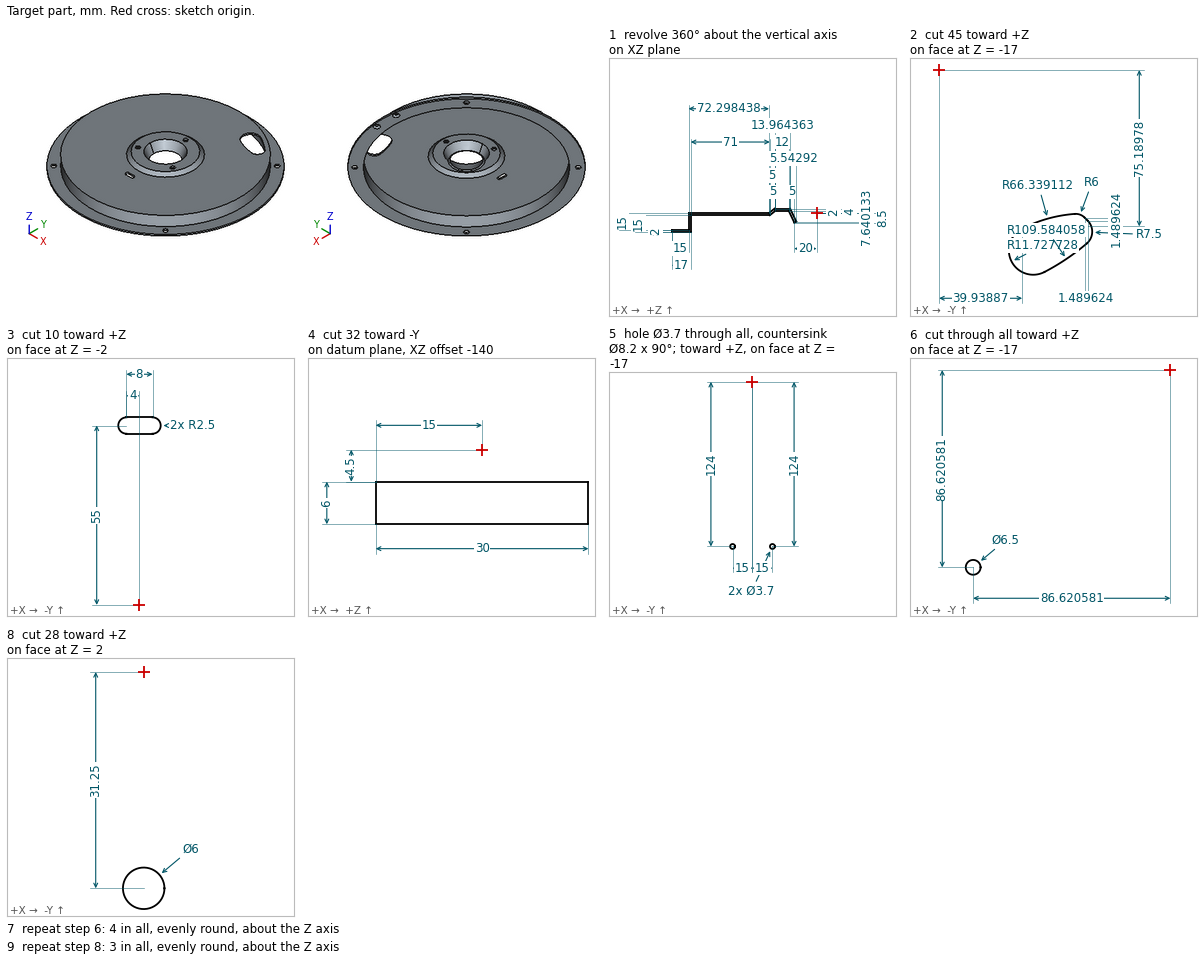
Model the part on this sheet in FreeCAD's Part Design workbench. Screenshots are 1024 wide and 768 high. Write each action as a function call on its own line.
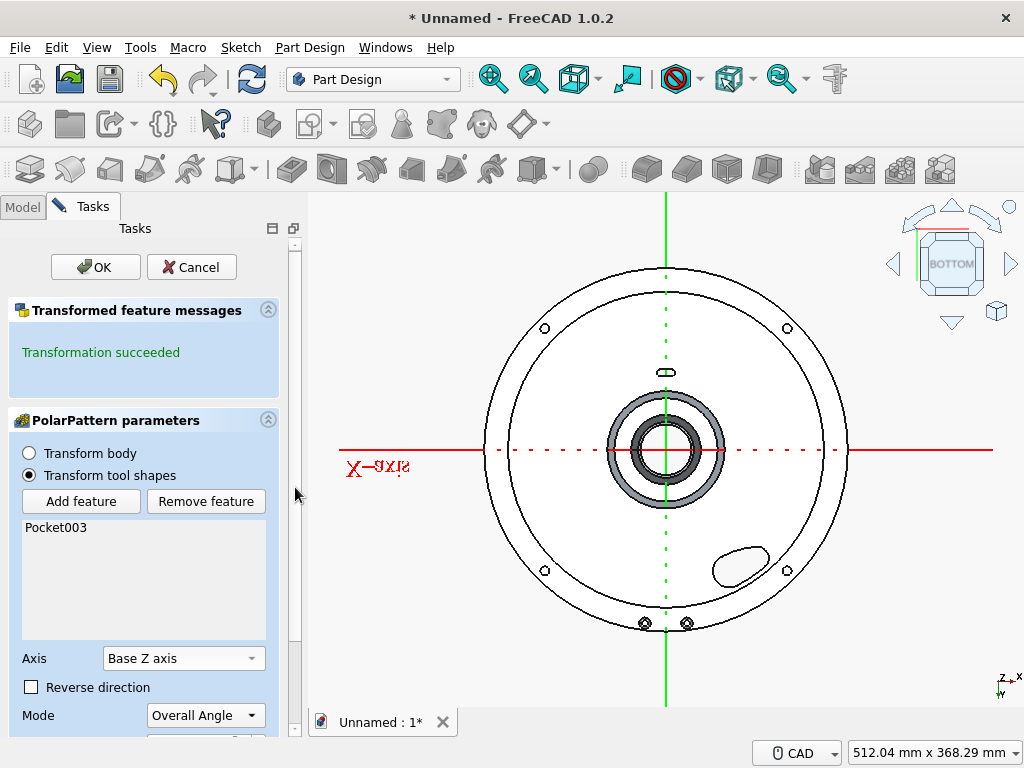
click(96, 267)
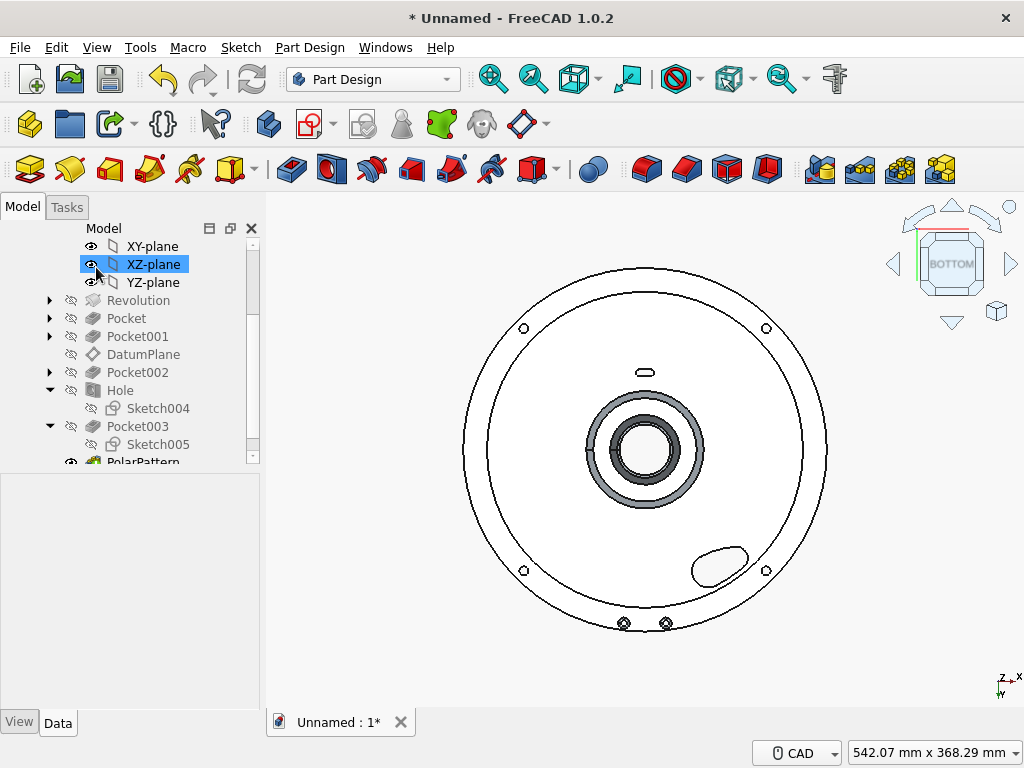
click(645, 493)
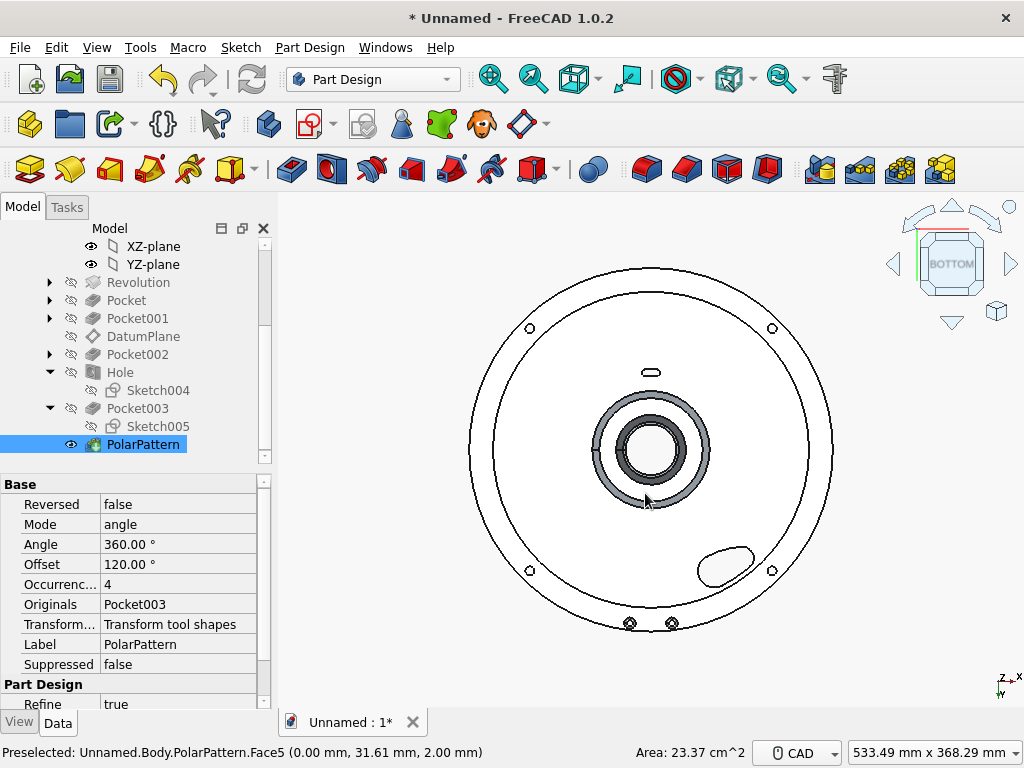
click(310, 124)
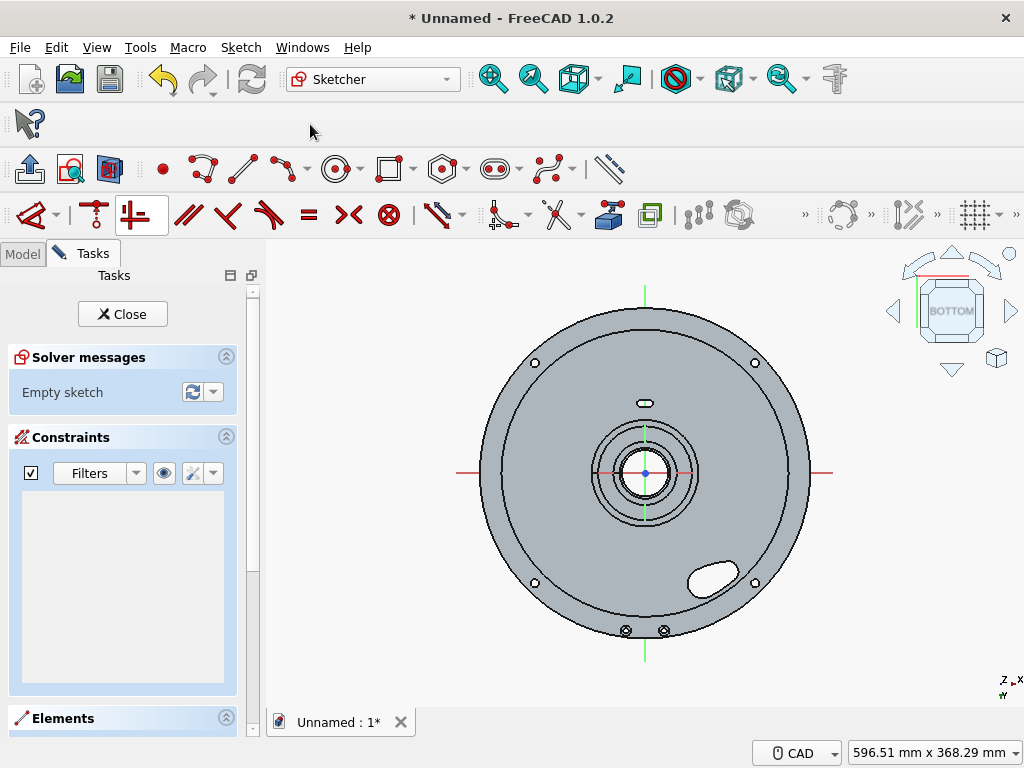
scroll(649, 515, up, 15)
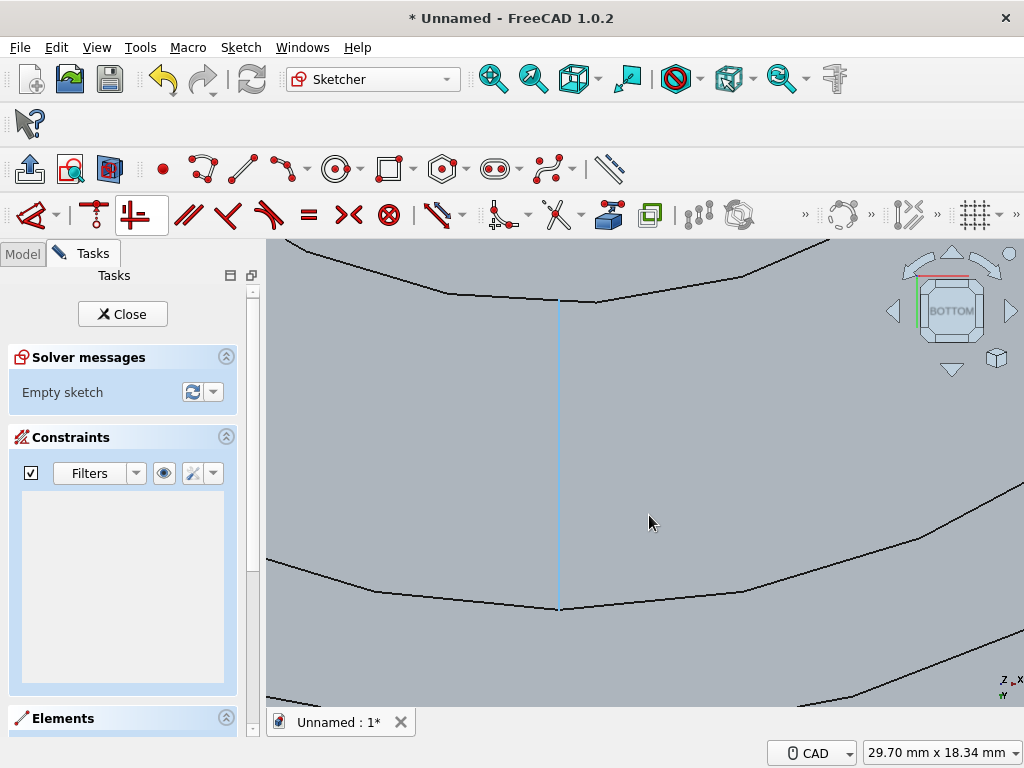
scroll(538, 451, up, 3)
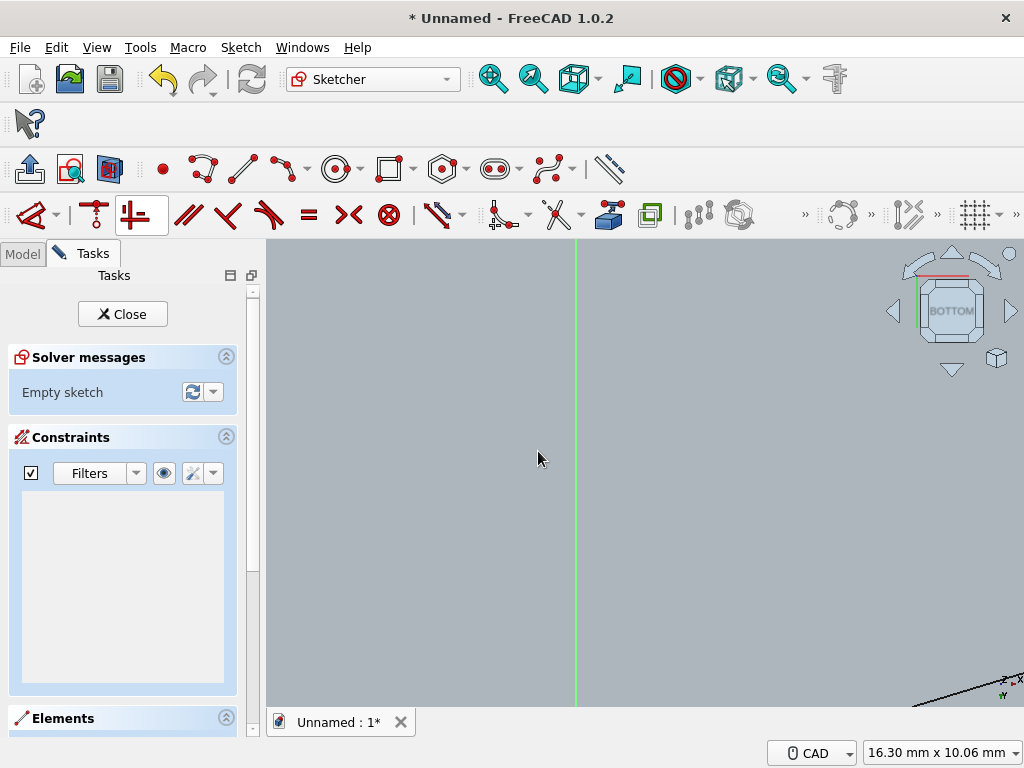
click(336, 170)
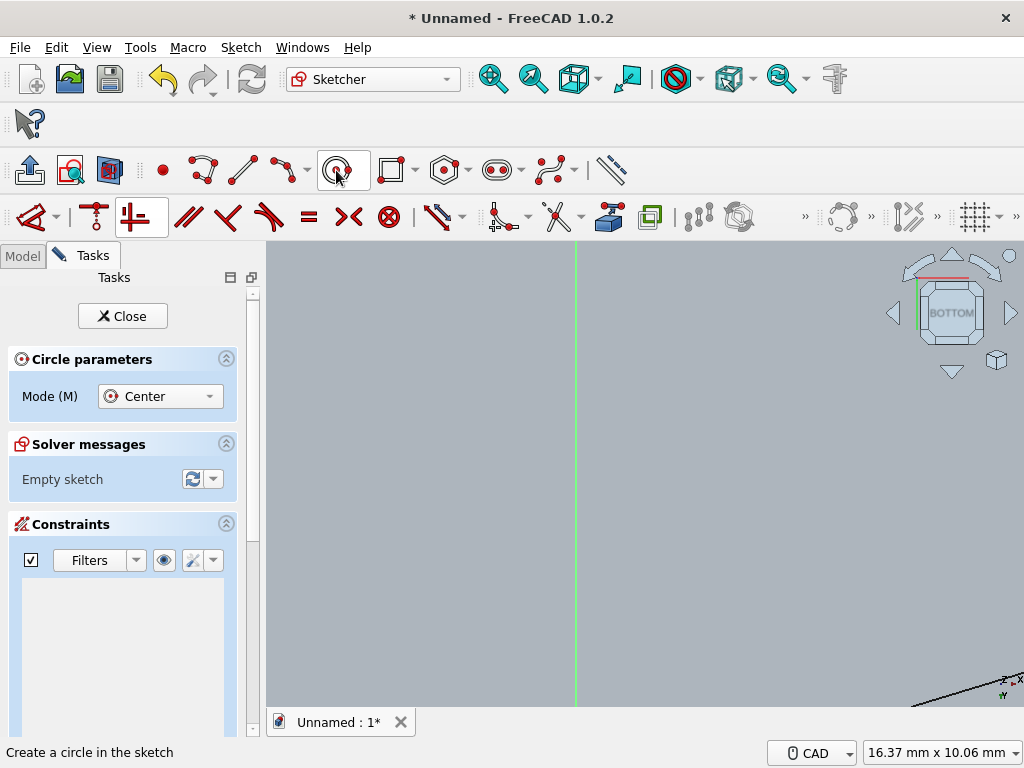
click(576, 474)
click(675, 376)
key(Escape)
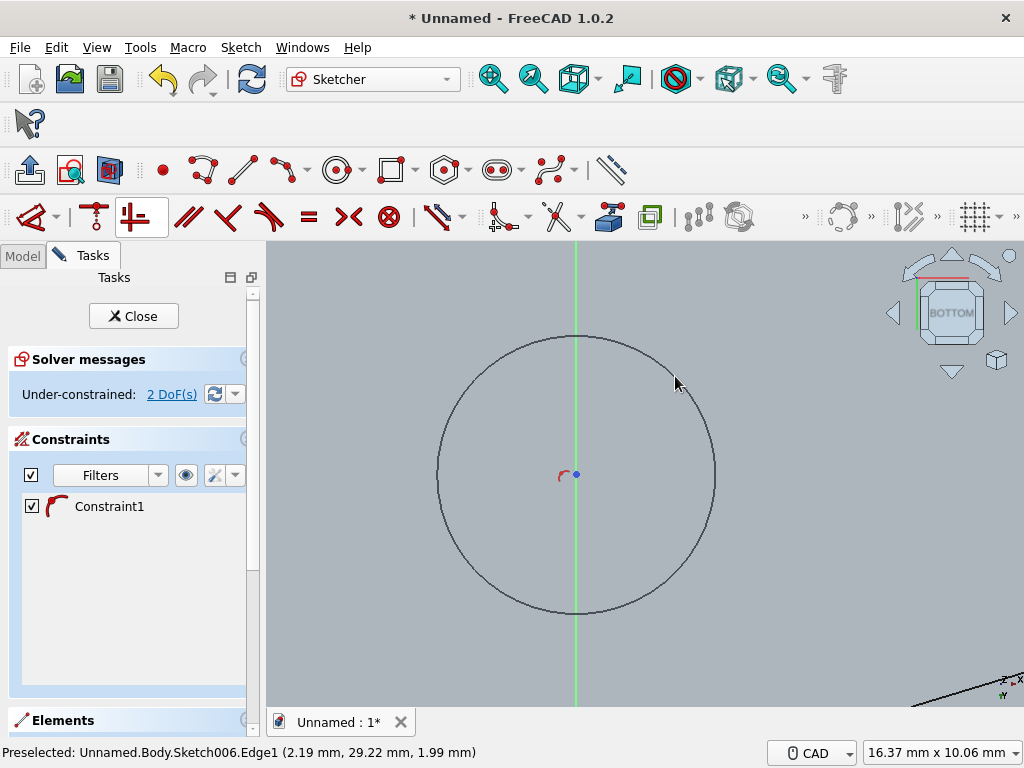
click(32, 218)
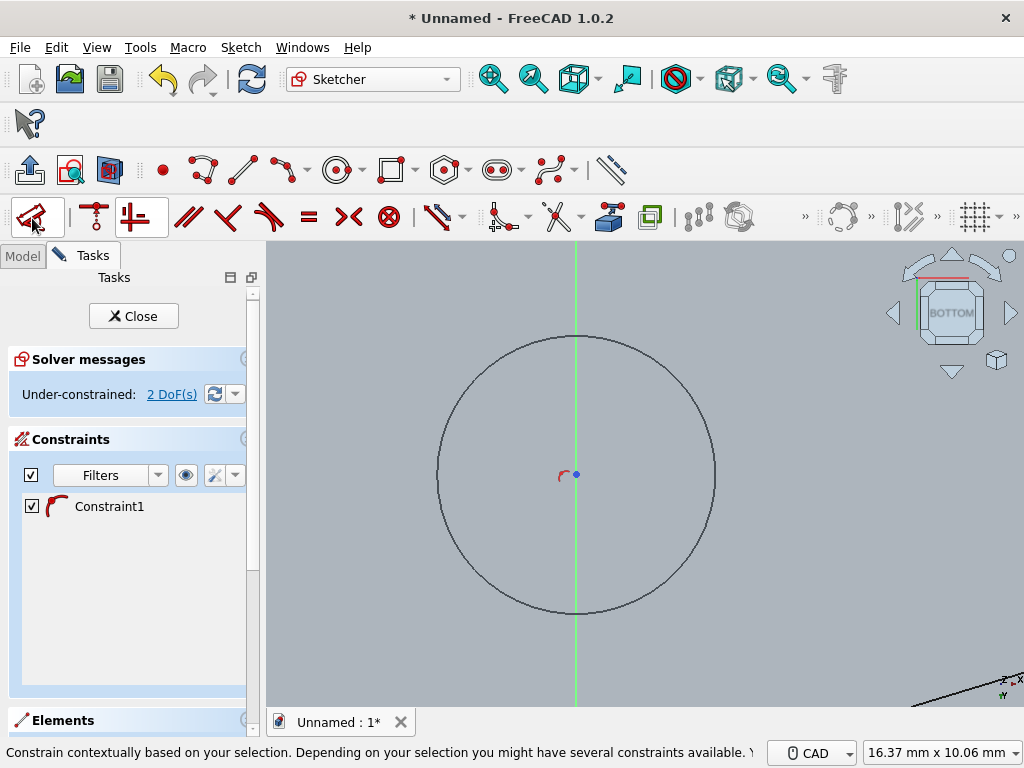
click(674, 376)
click(696, 353)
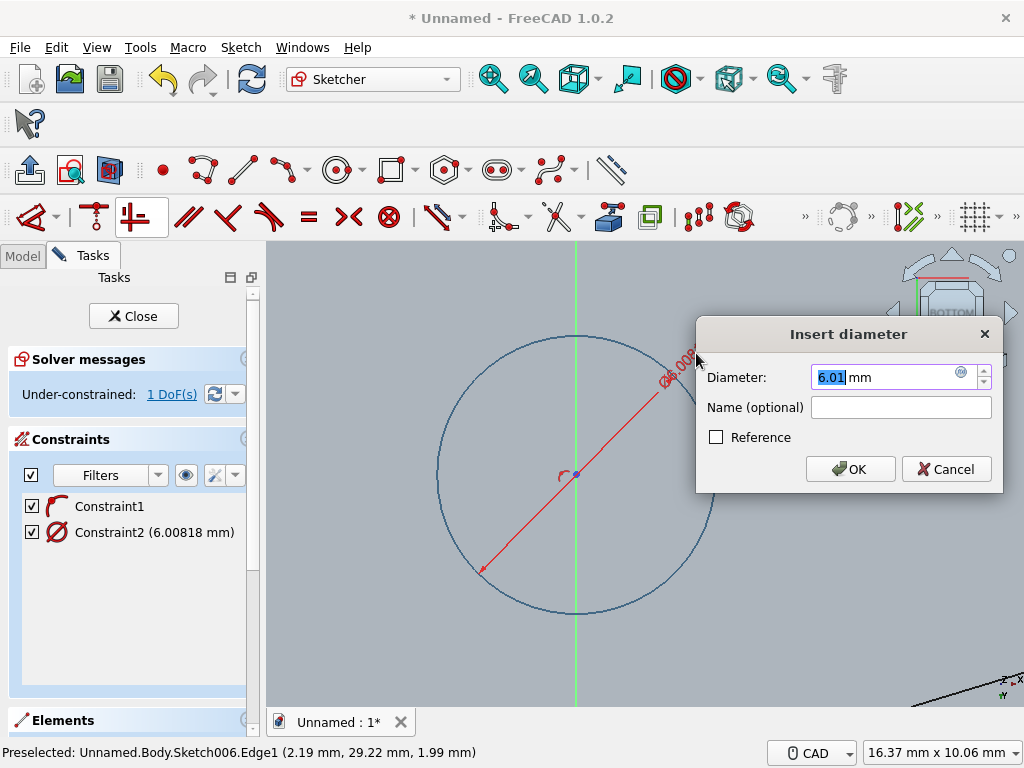
text(6)
key(Return)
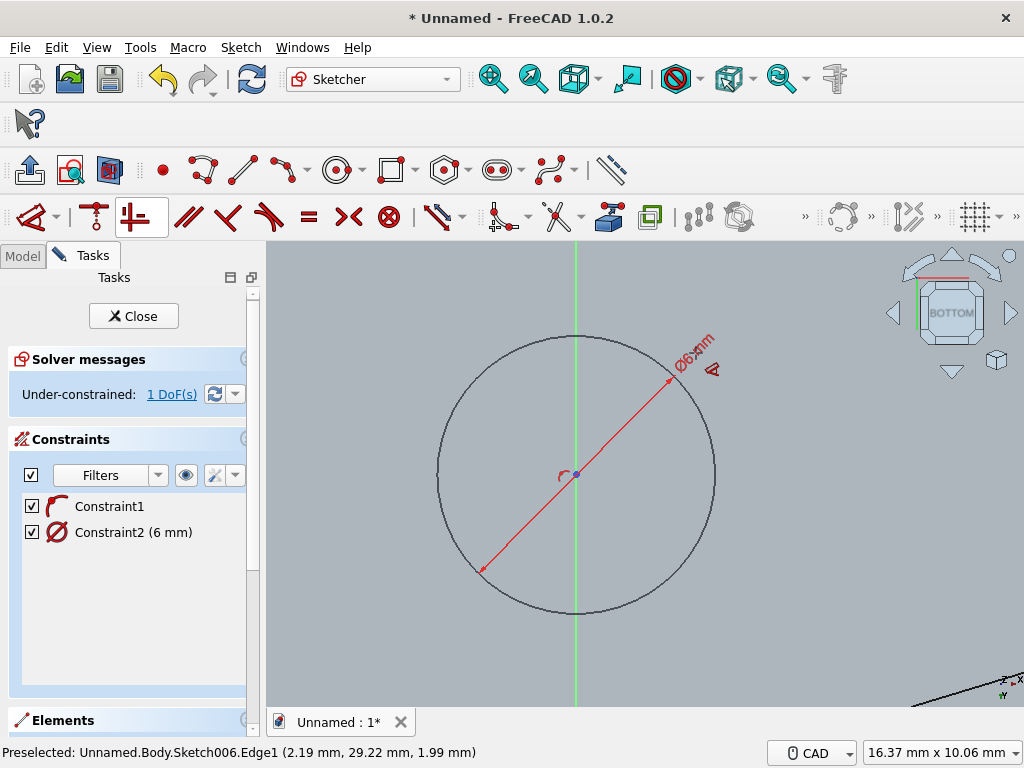
click(576, 475)
click(610, 372)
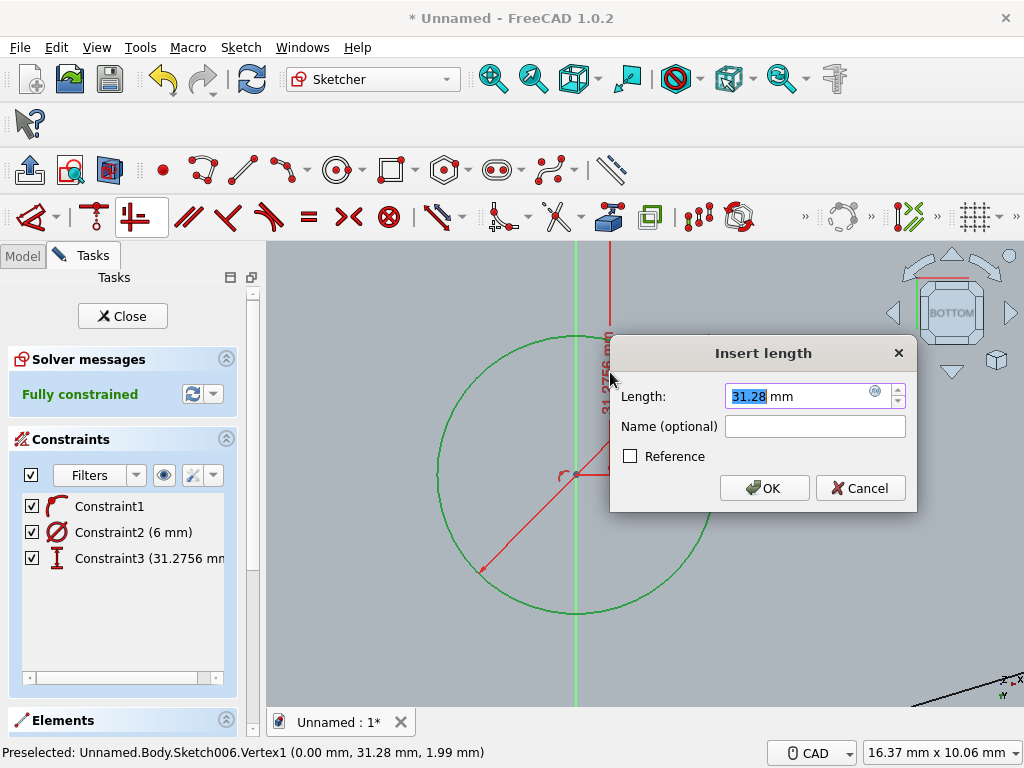
text(31.25)
key(Return)
key(Escape)